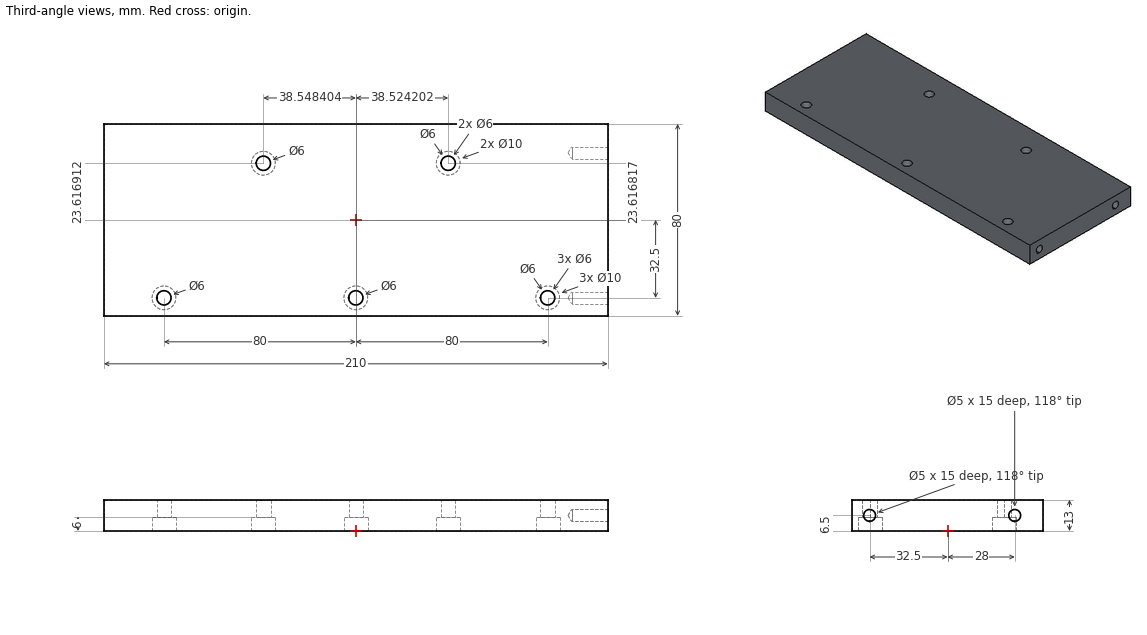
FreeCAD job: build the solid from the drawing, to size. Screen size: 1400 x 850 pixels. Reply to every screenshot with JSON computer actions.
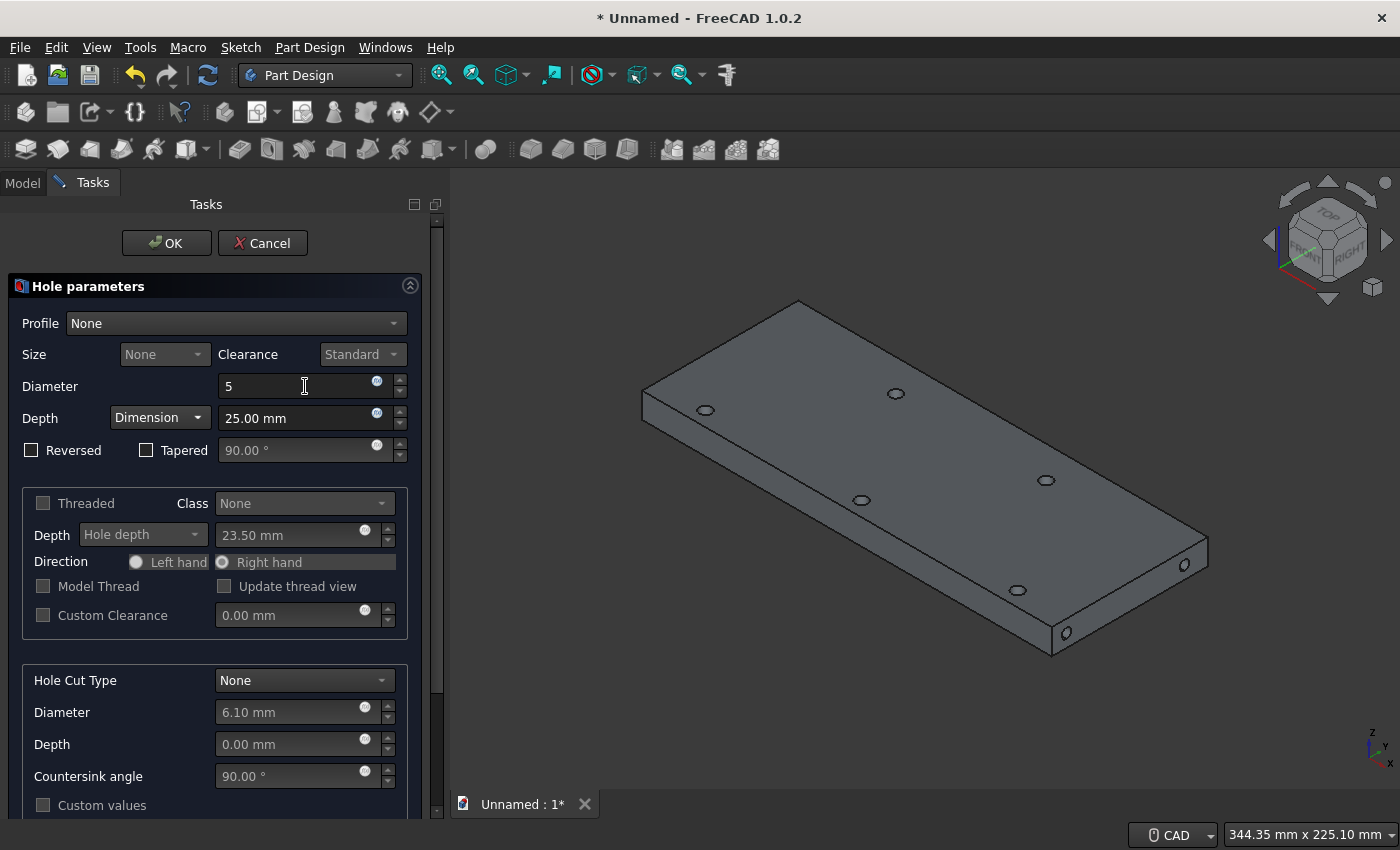
{"action": "triple_click", "coordinate": [305, 418]}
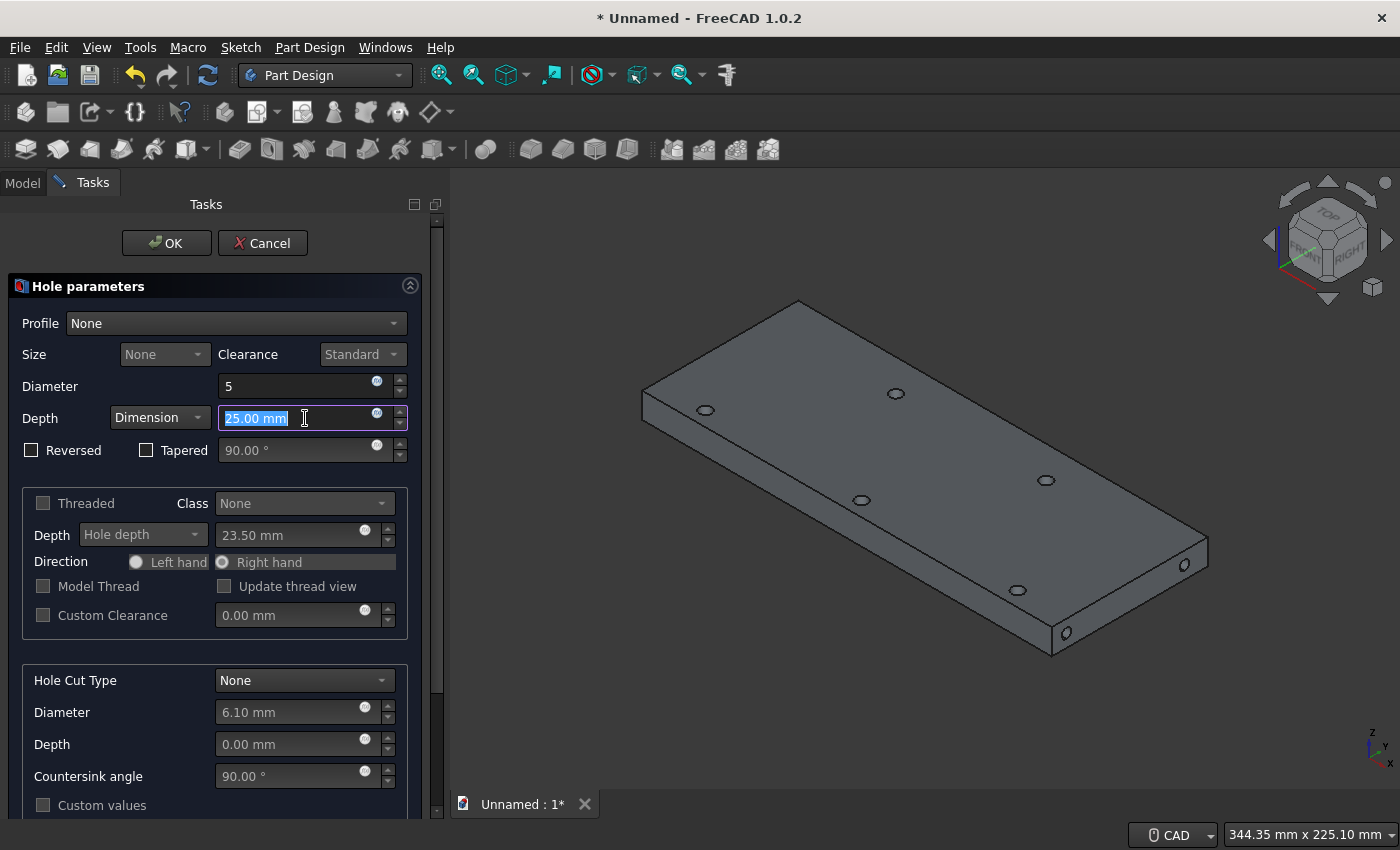
{"action": "type", "text": "15"}
{"action": "key", "text": "Tab"}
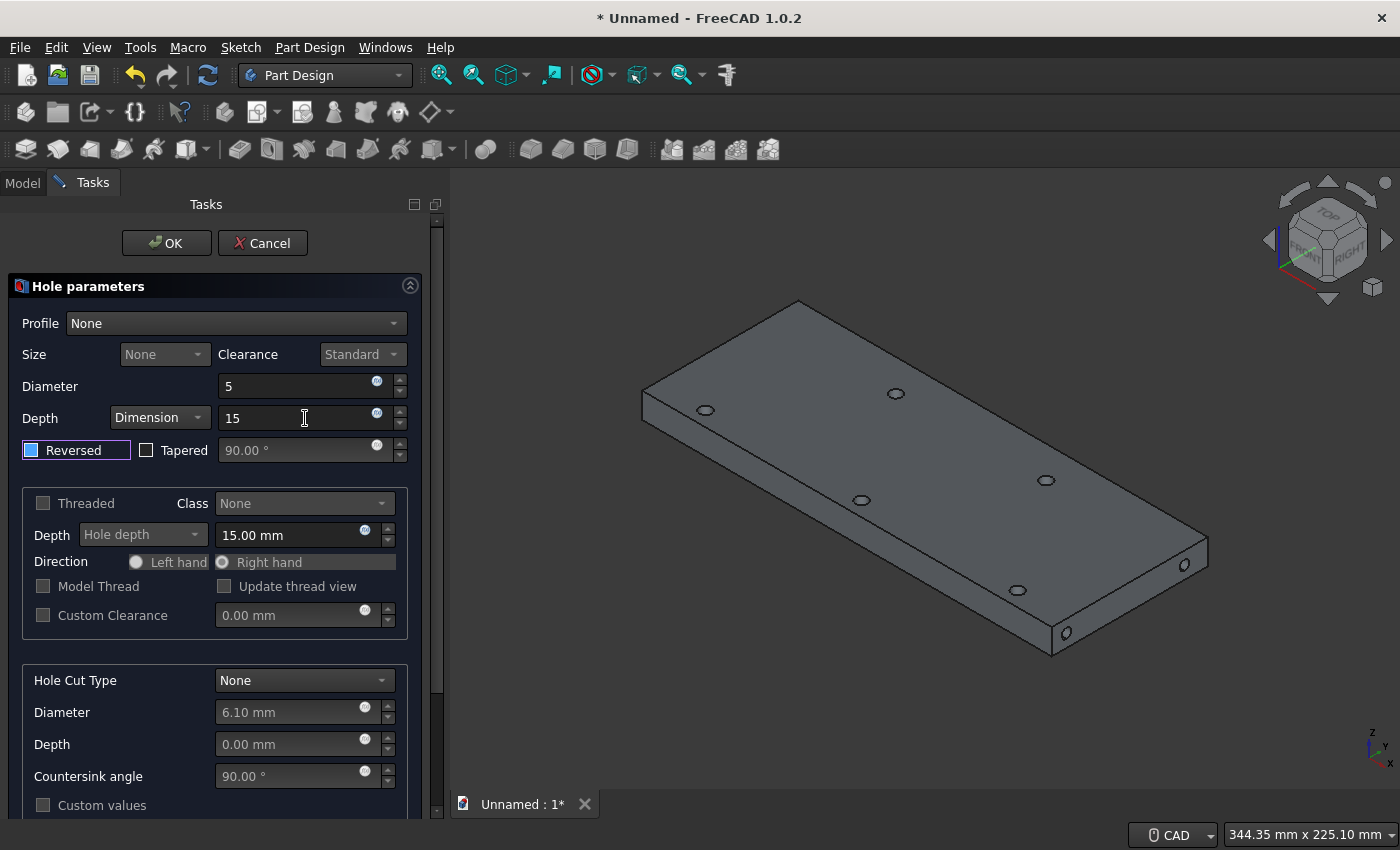
{"action": "left_click", "coordinate": [167, 243]}